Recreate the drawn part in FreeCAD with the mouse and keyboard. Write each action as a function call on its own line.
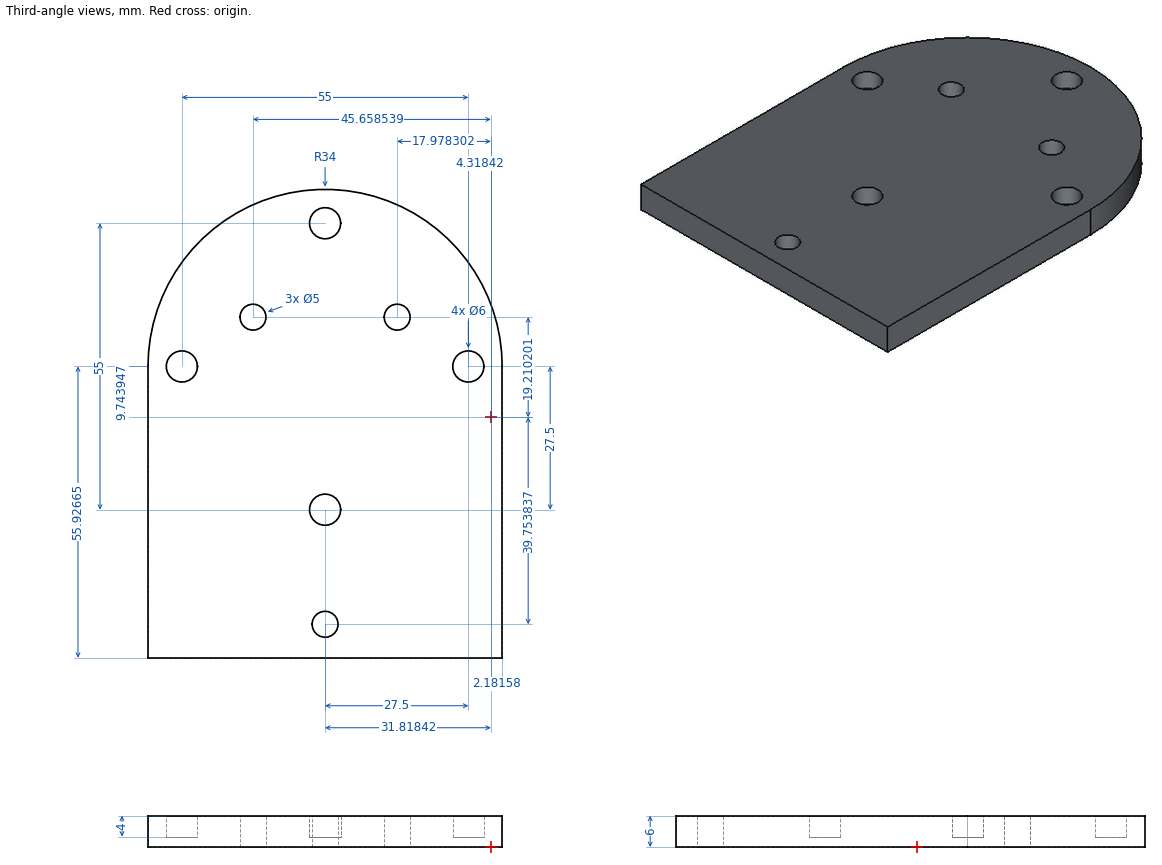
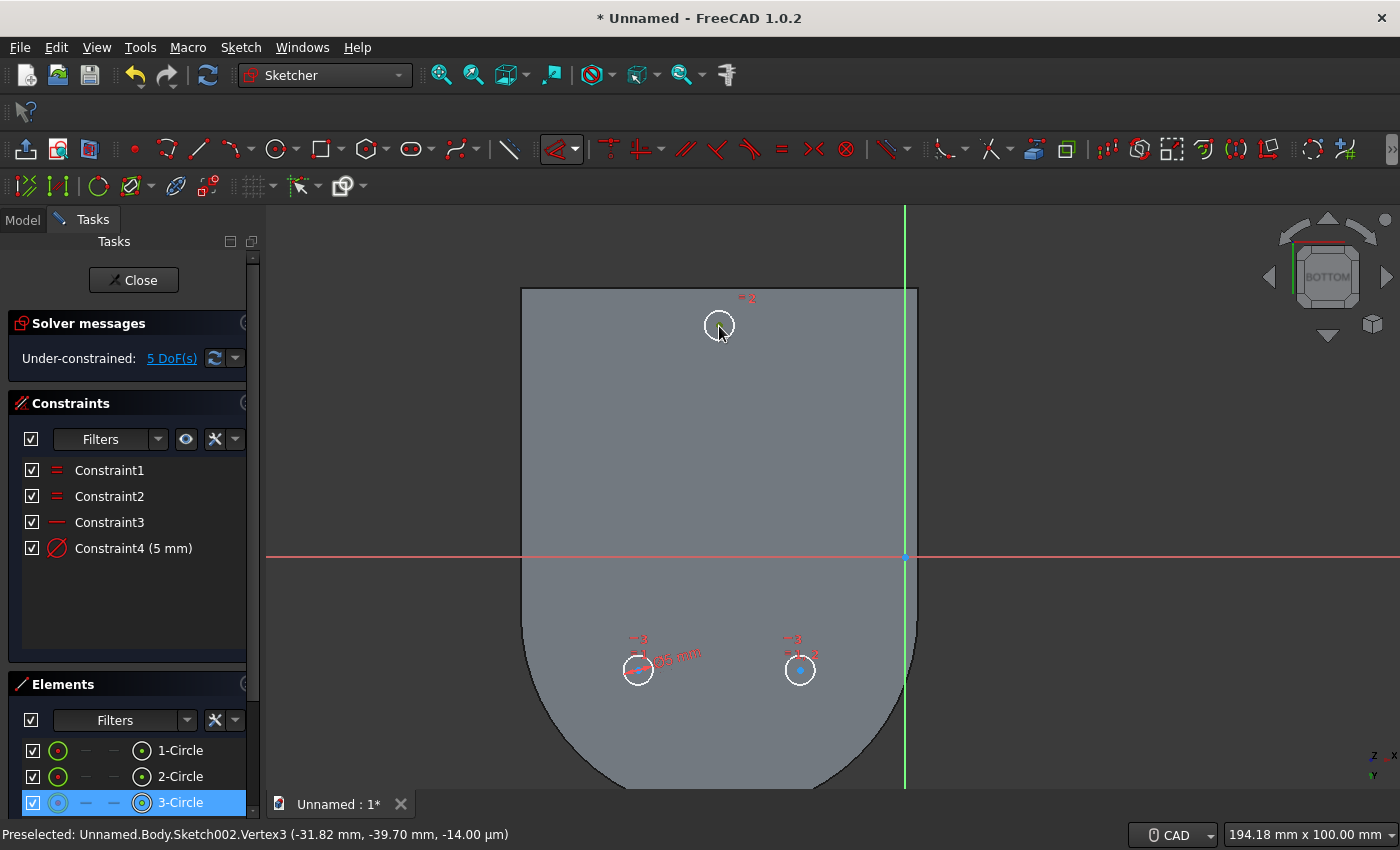
key(l)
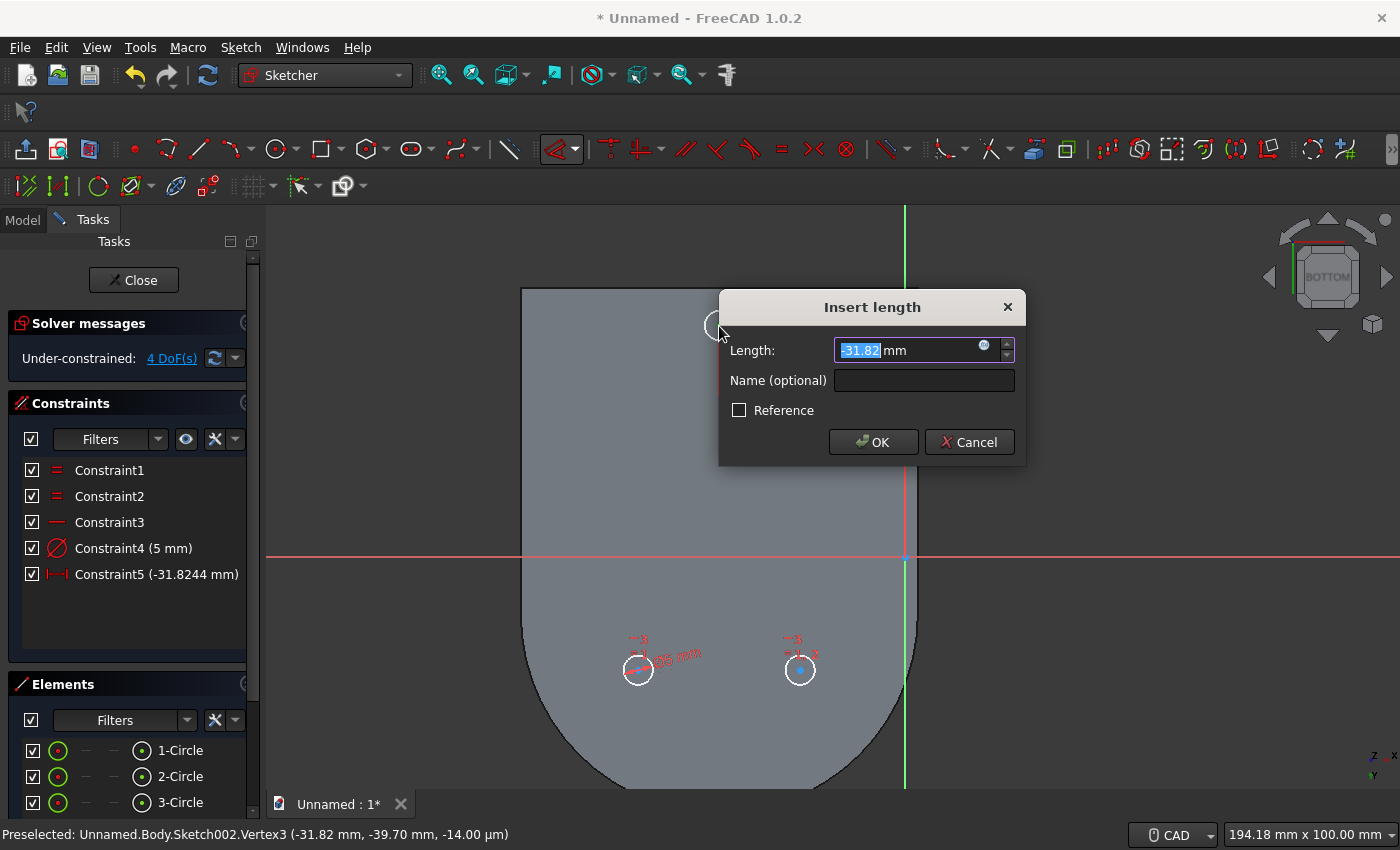
text(-31.81842)
key(Return)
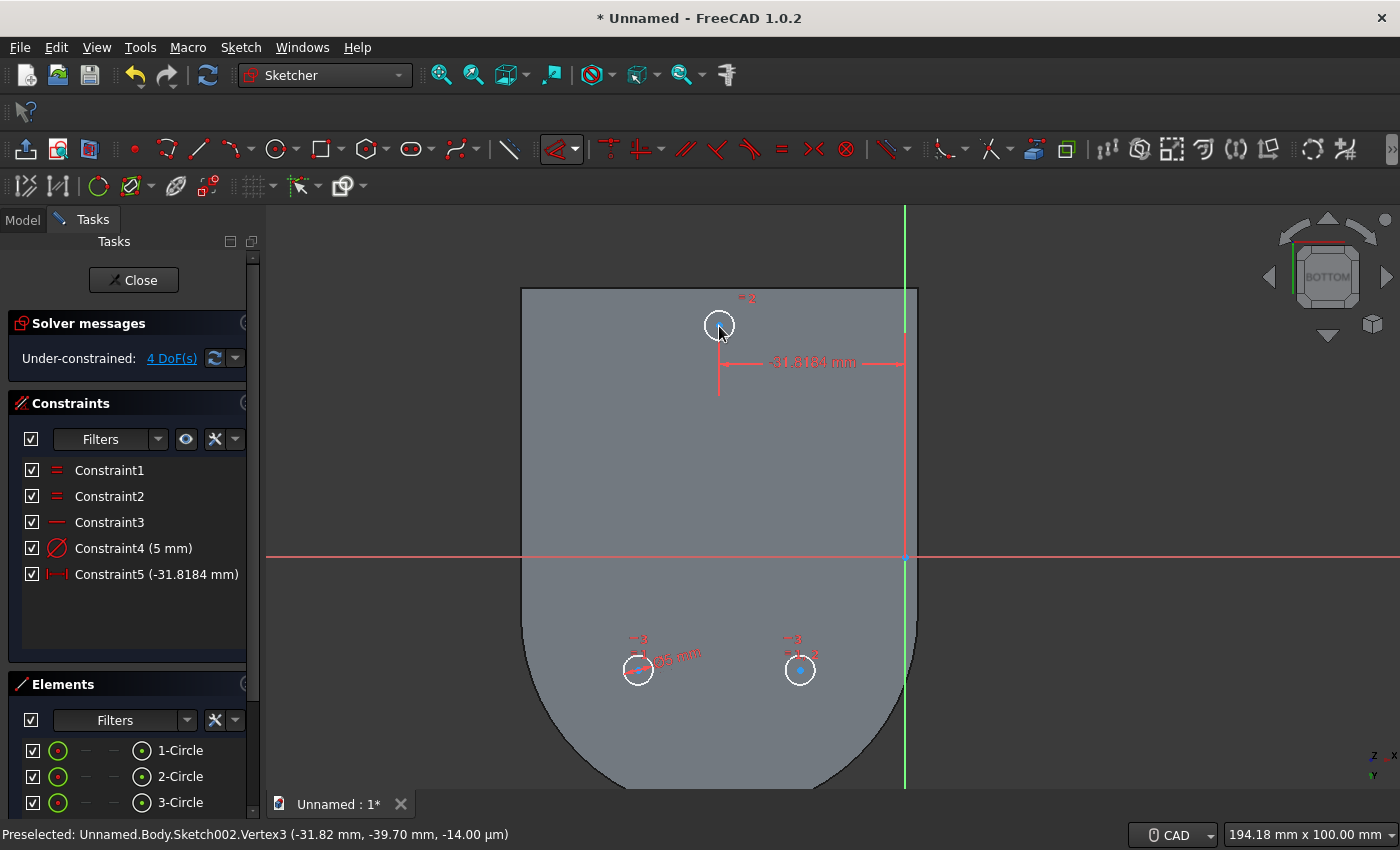
click(638, 670)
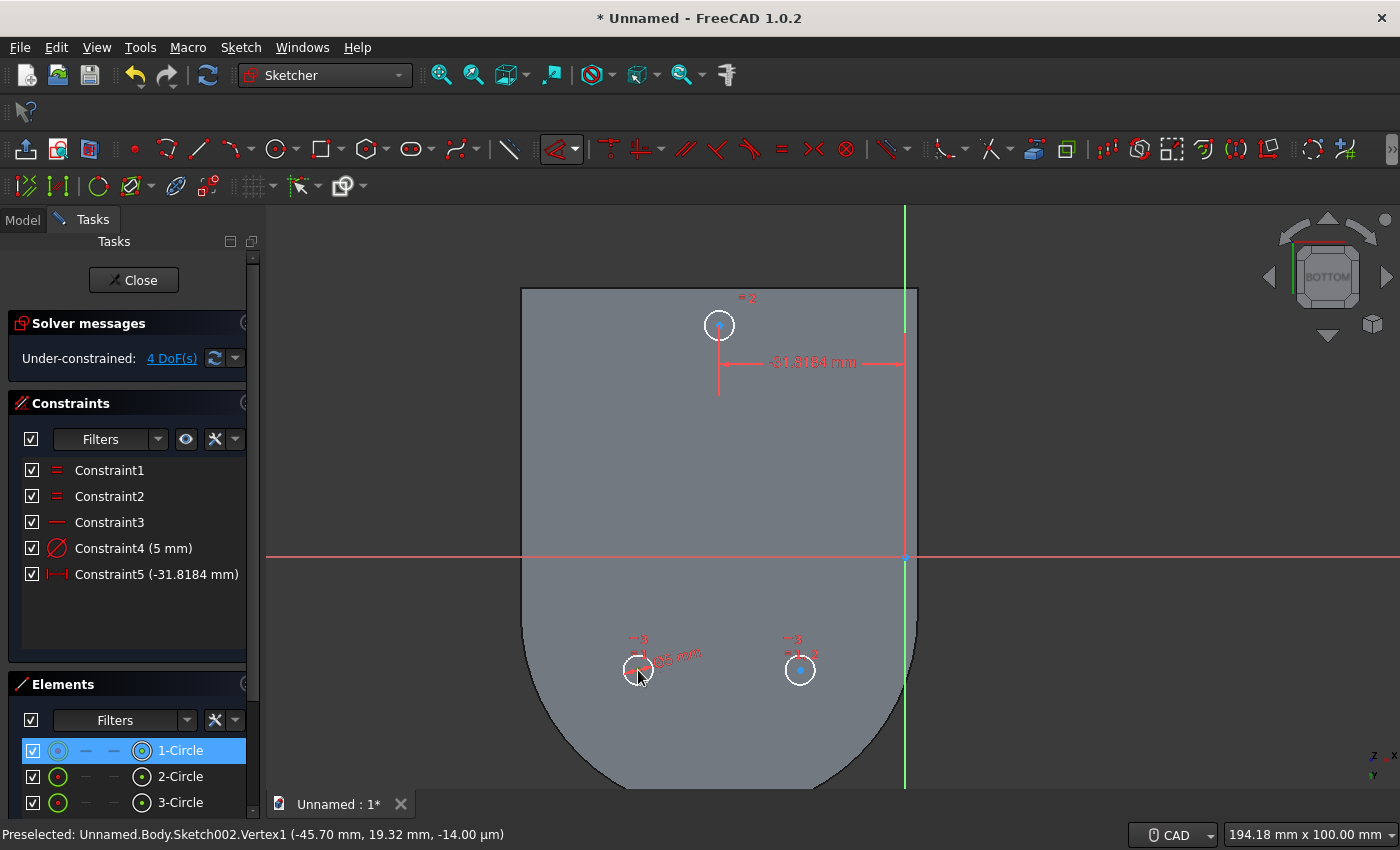
click(578, 150)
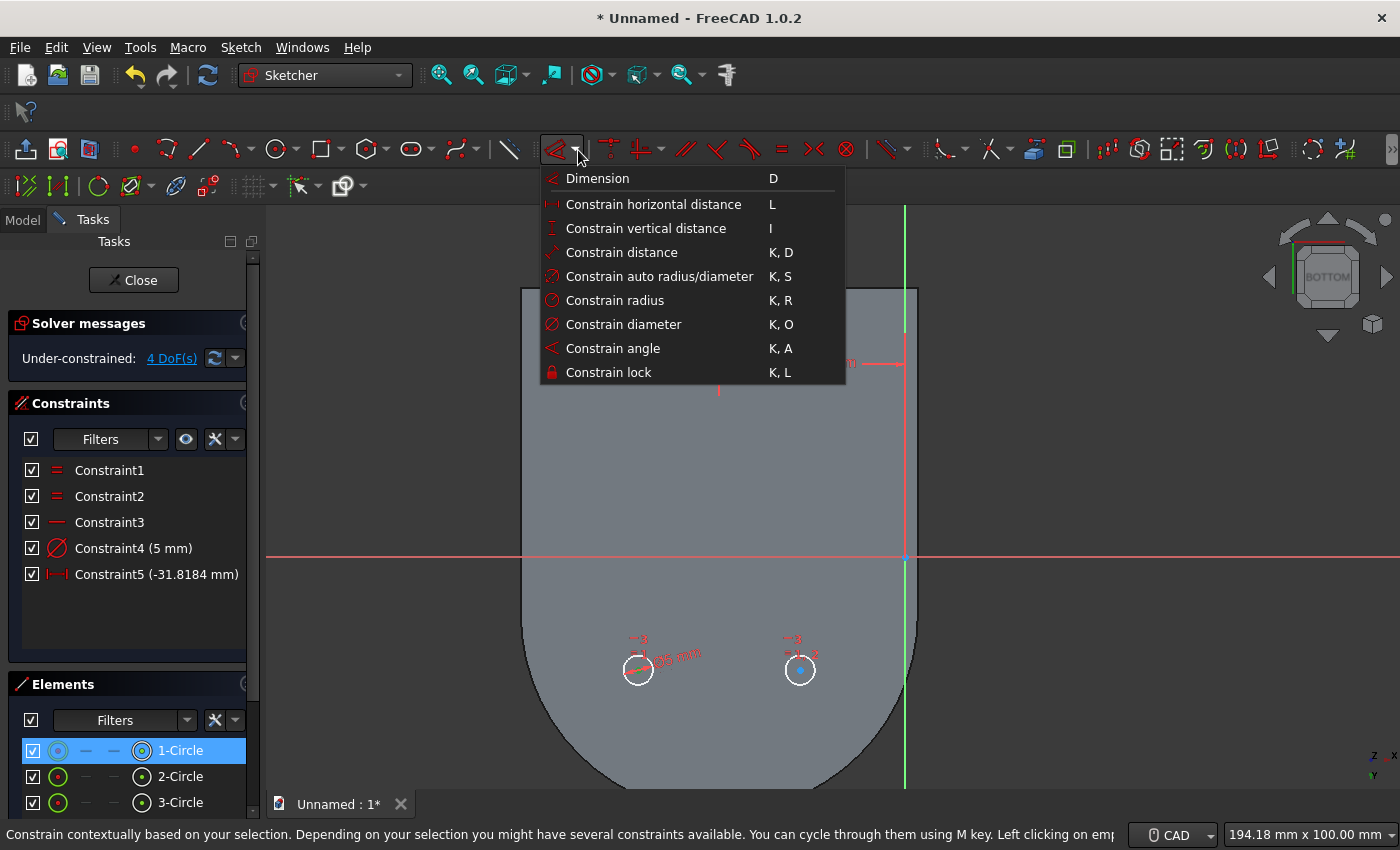
click(693, 204)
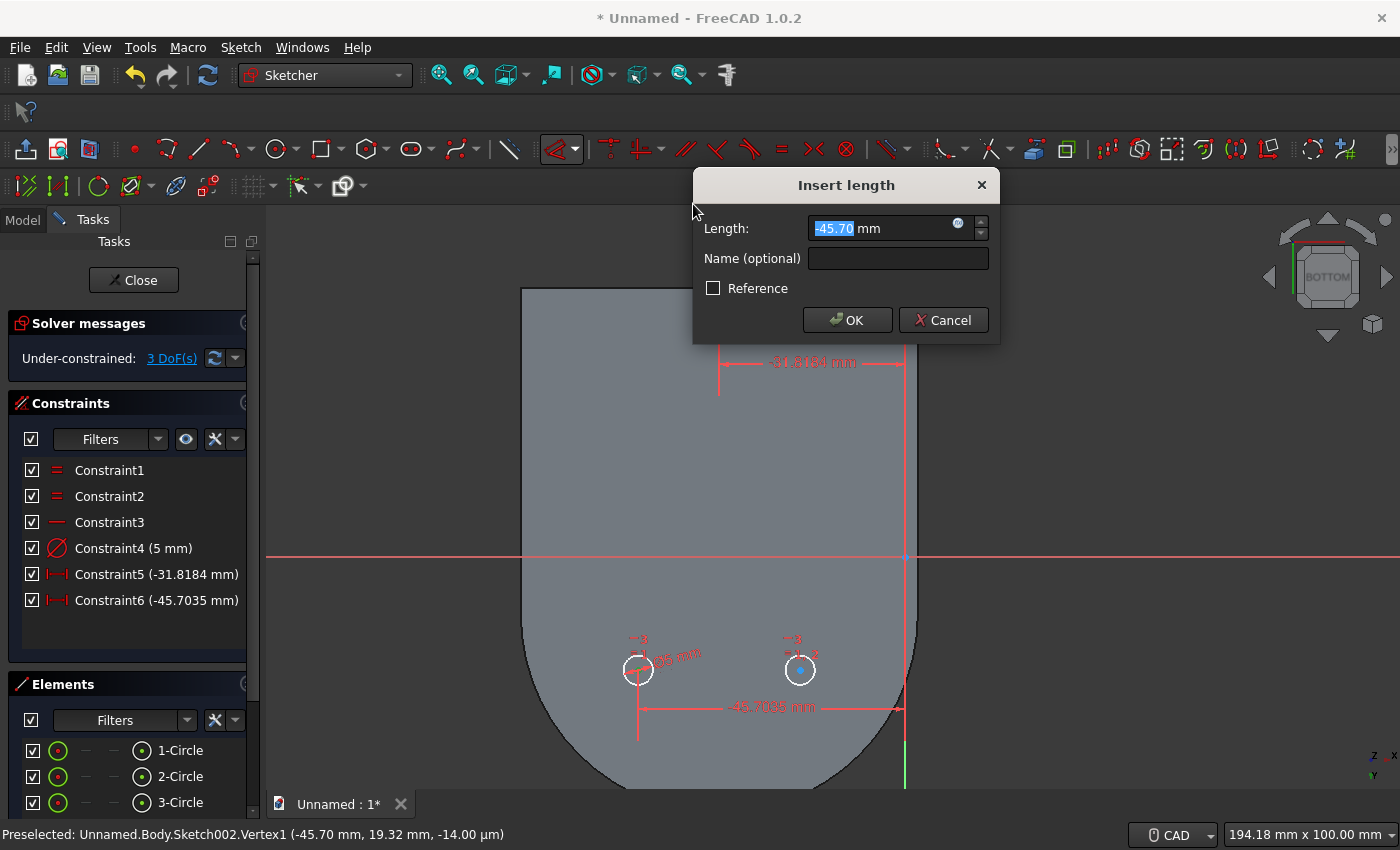
text(-45.658539)
key(Return)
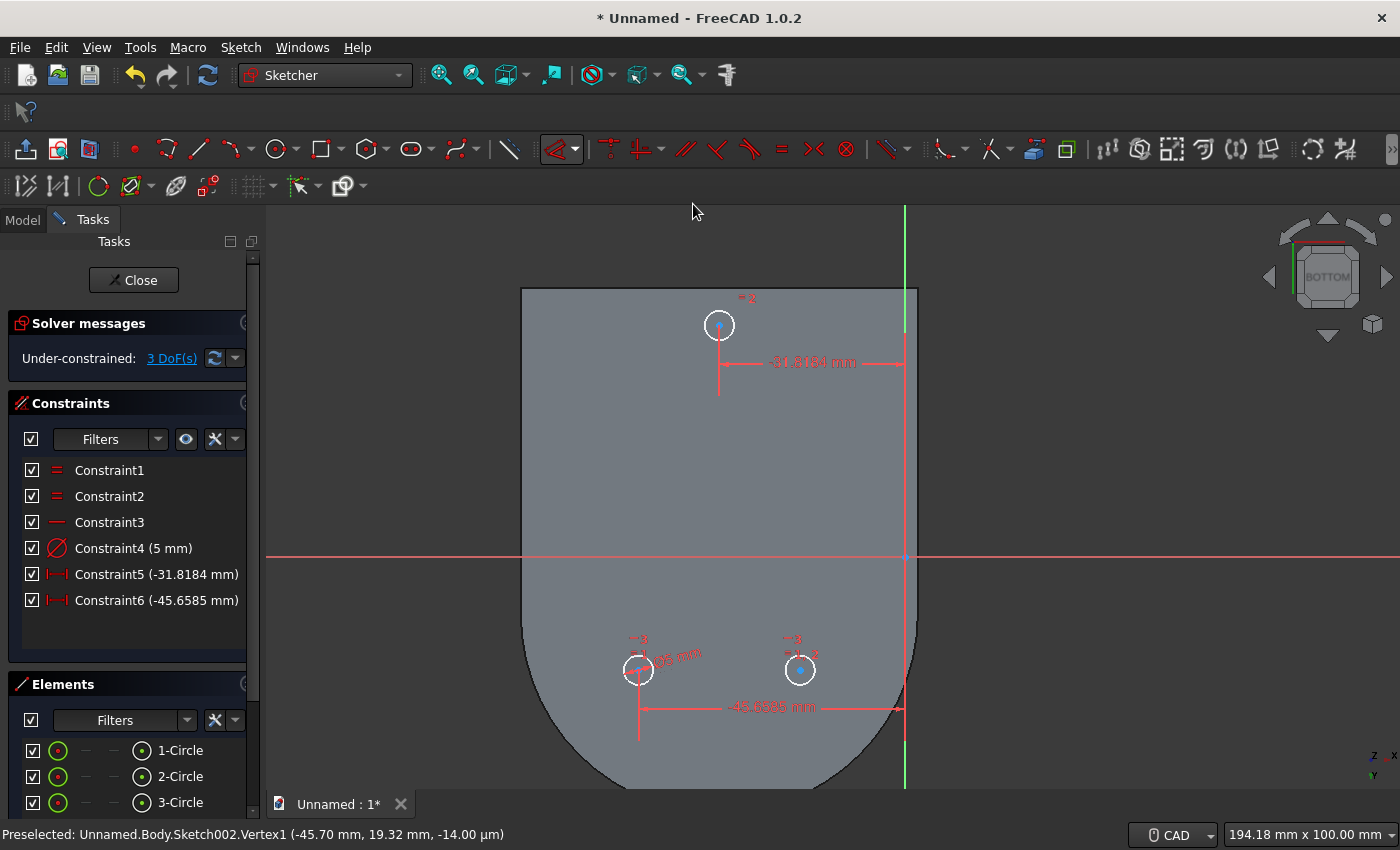
click(639, 670)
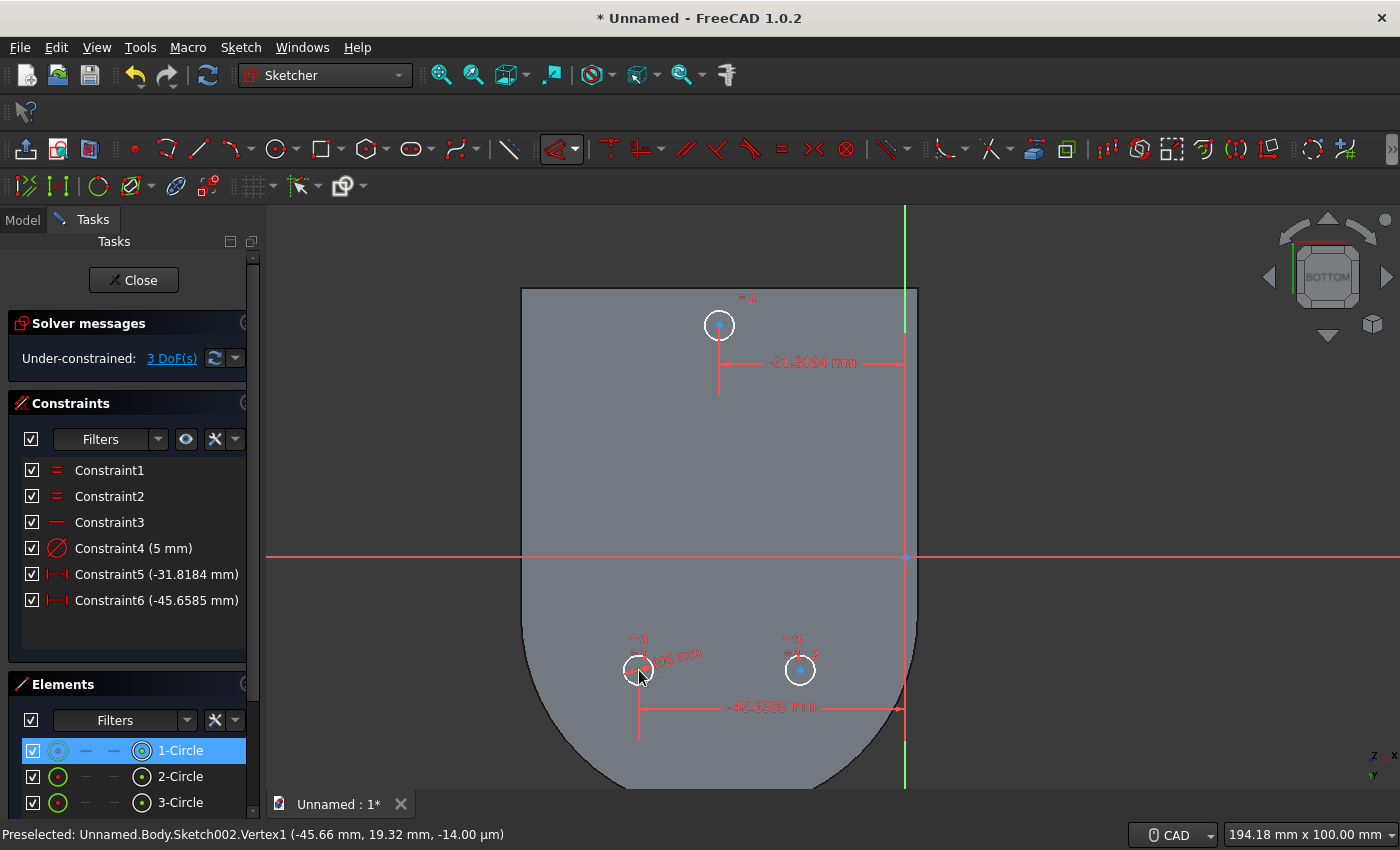
key(i)